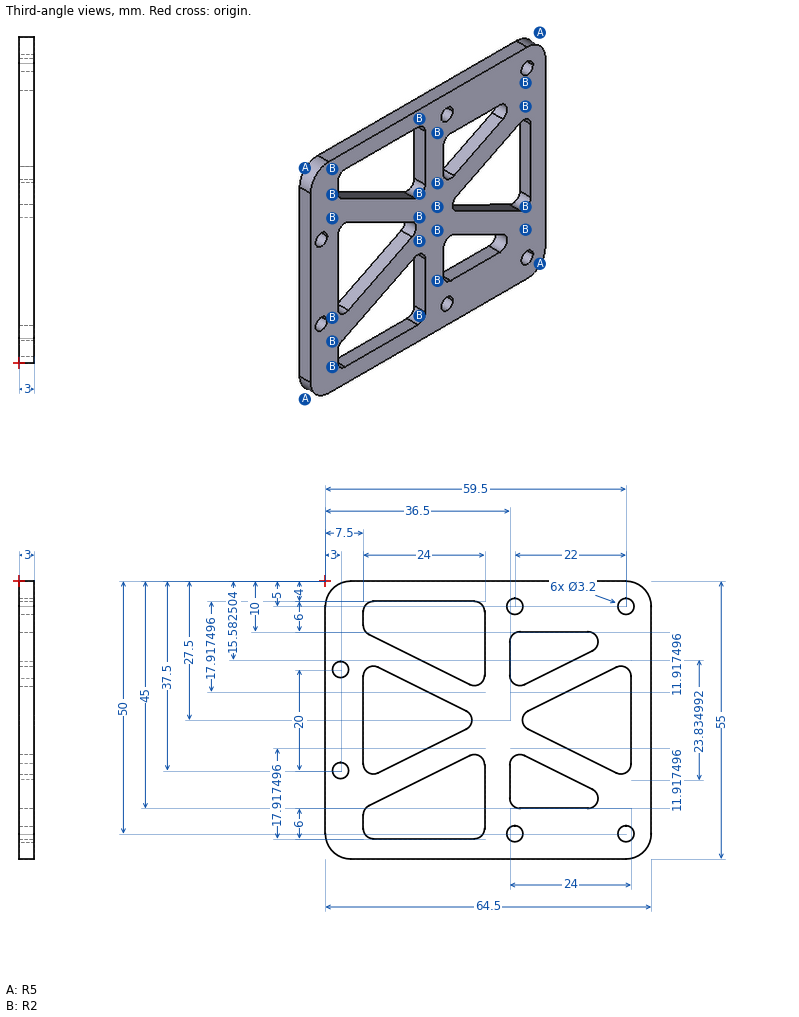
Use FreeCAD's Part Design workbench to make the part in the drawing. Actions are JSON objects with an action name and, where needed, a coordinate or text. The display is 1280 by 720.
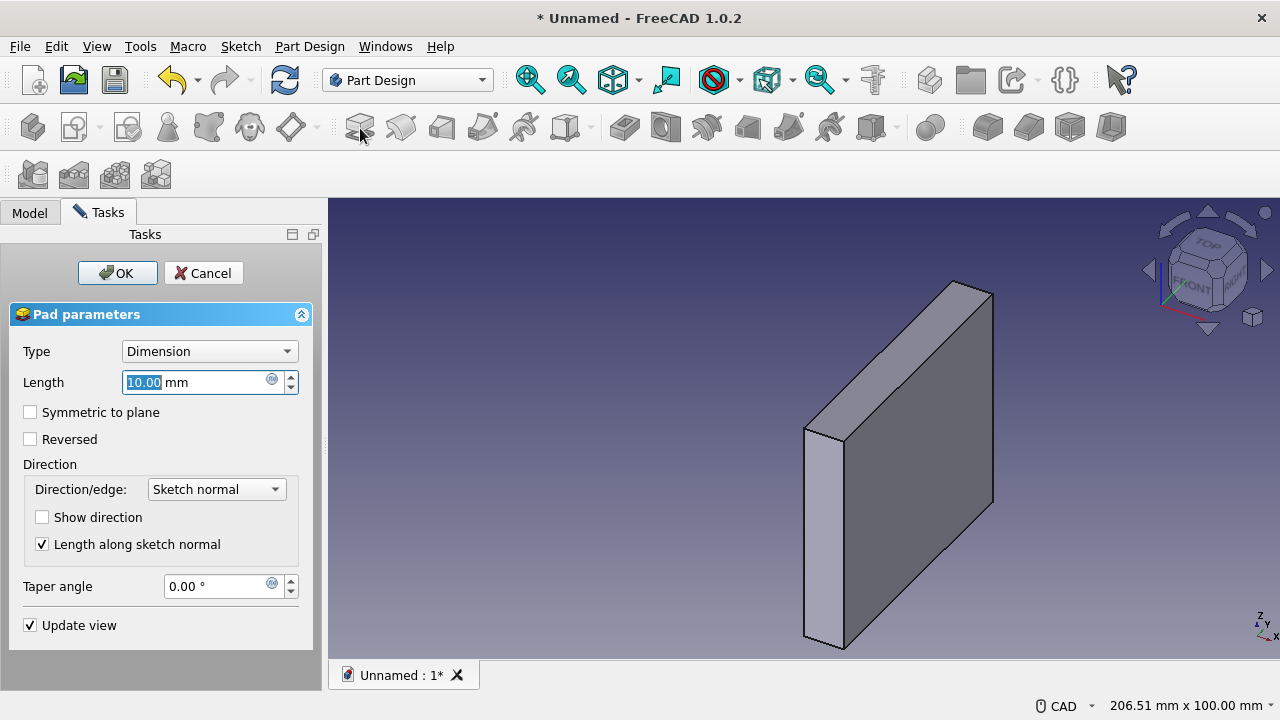
{"action": "type", "text": "3"}
{"action": "key", "text": "Tab"}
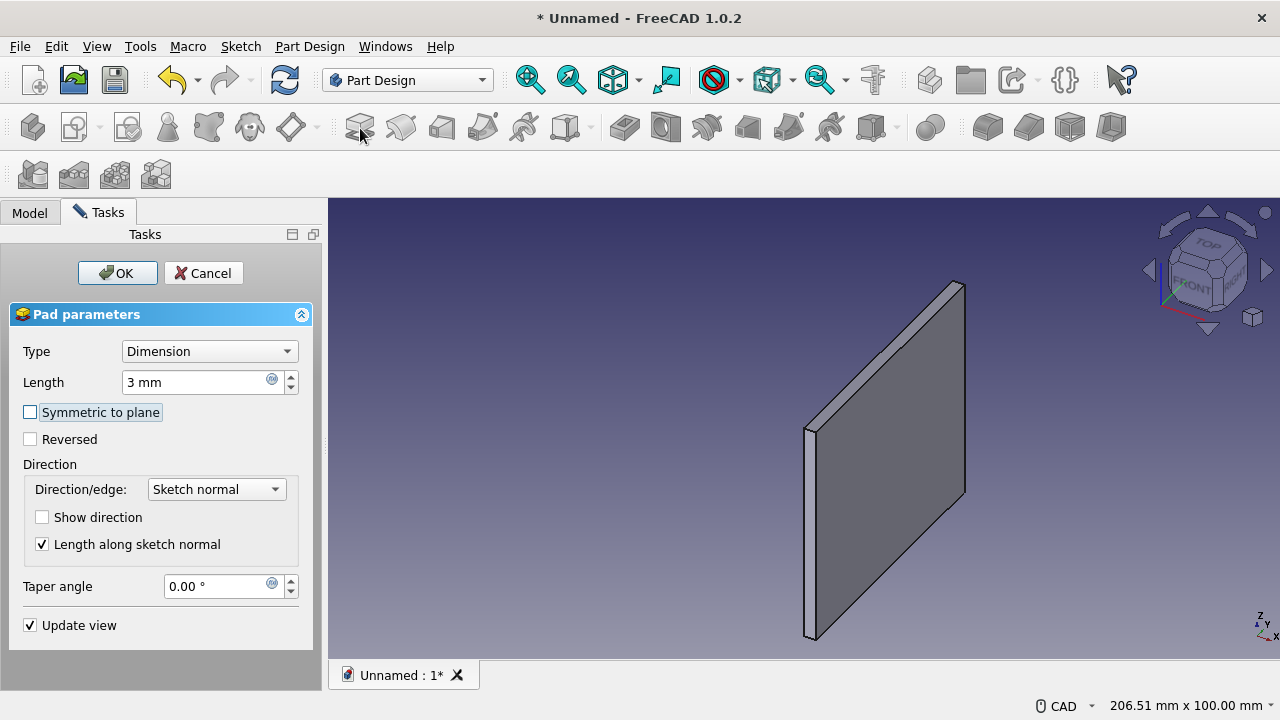
{"action": "left_click", "coordinate": [118, 273]}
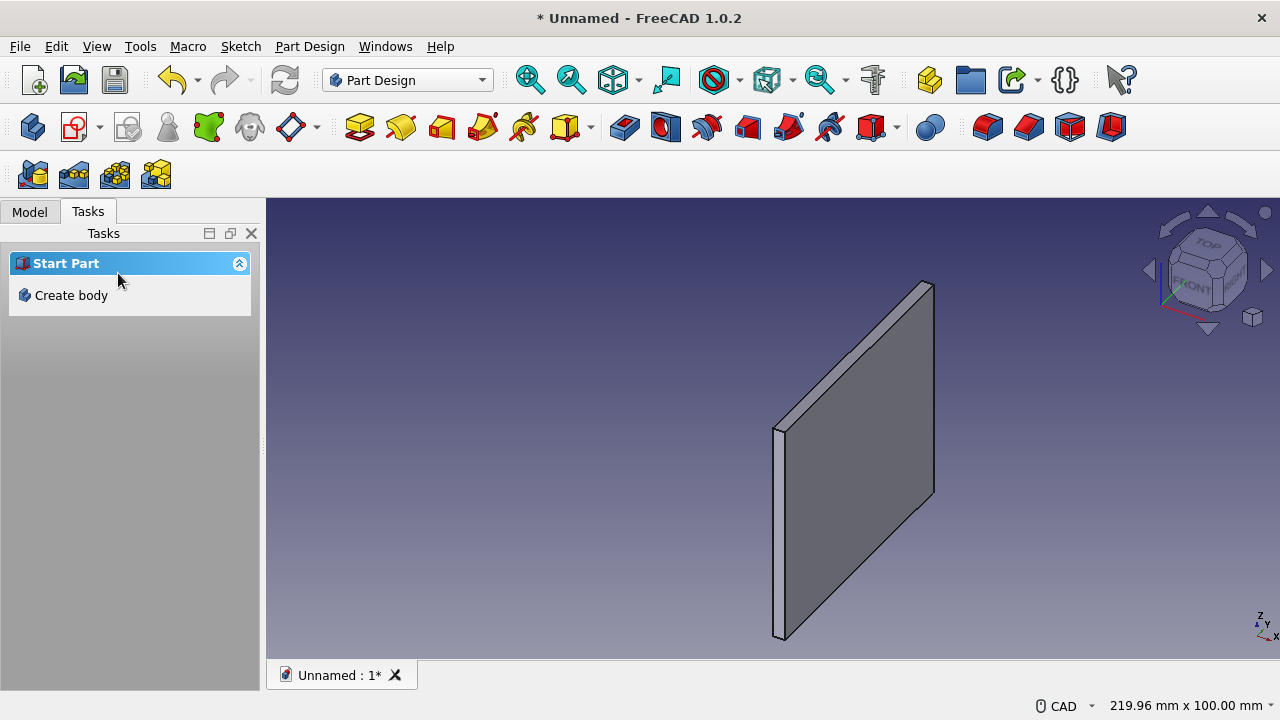
{"action": "left_click", "coordinate": [74, 128]}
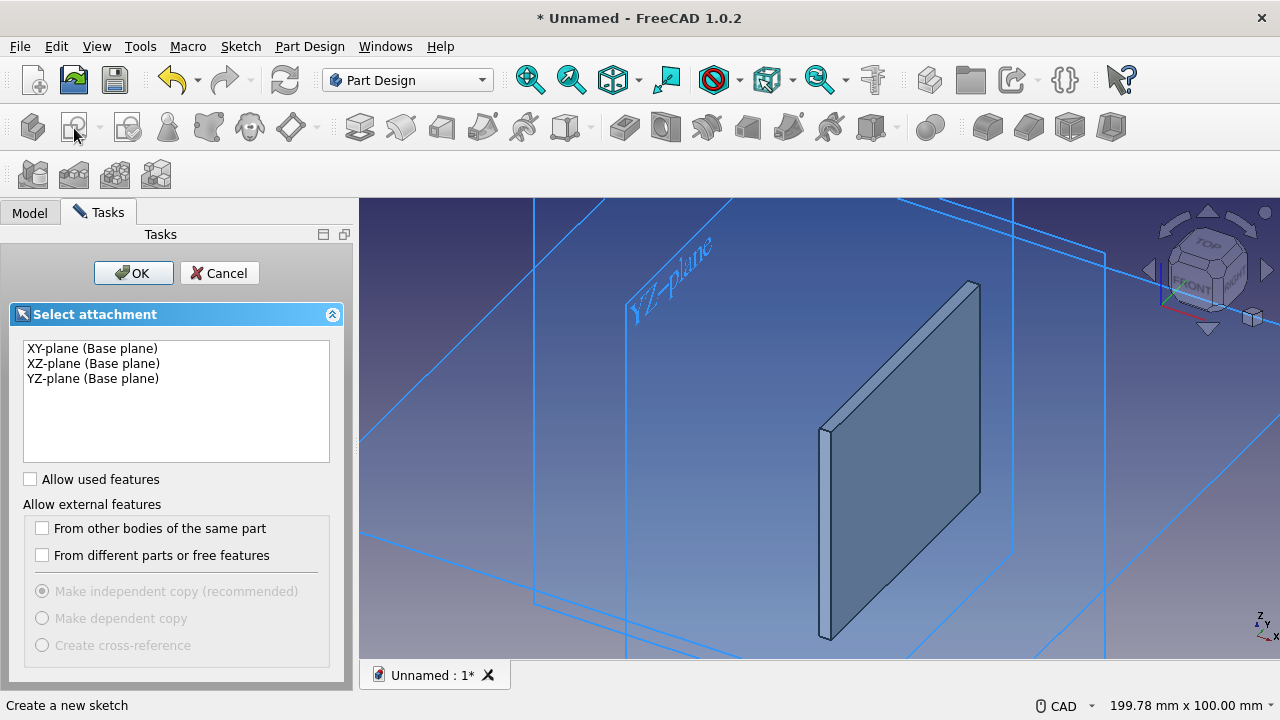
{"action": "left_click", "coordinate": [84, 378]}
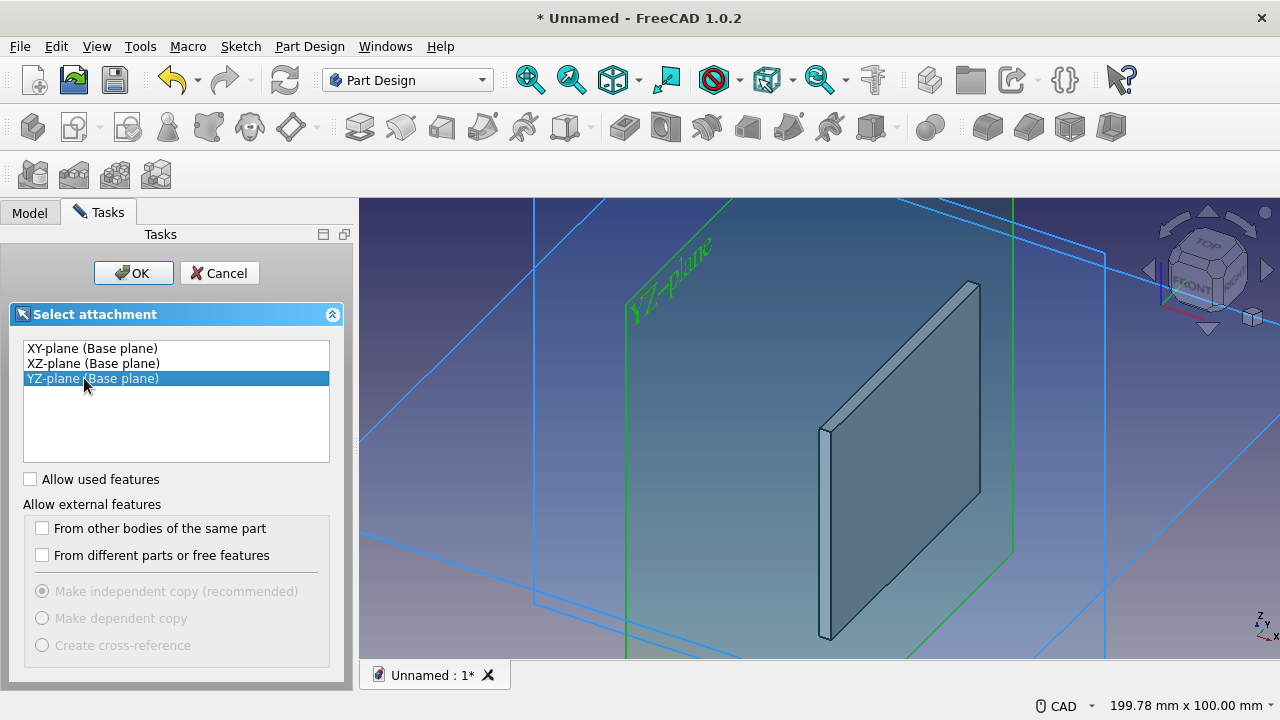
{"action": "left_click", "coordinate": [134, 273]}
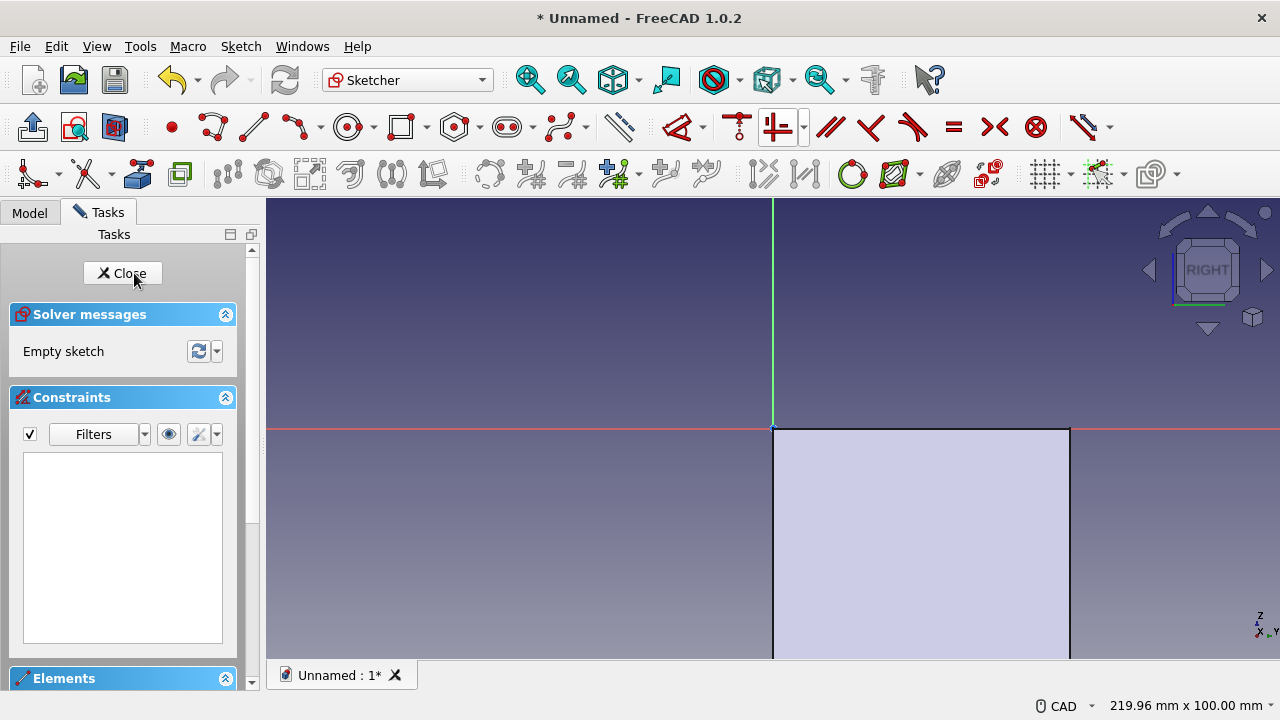
{"action": "left_click", "coordinate": [115, 128]}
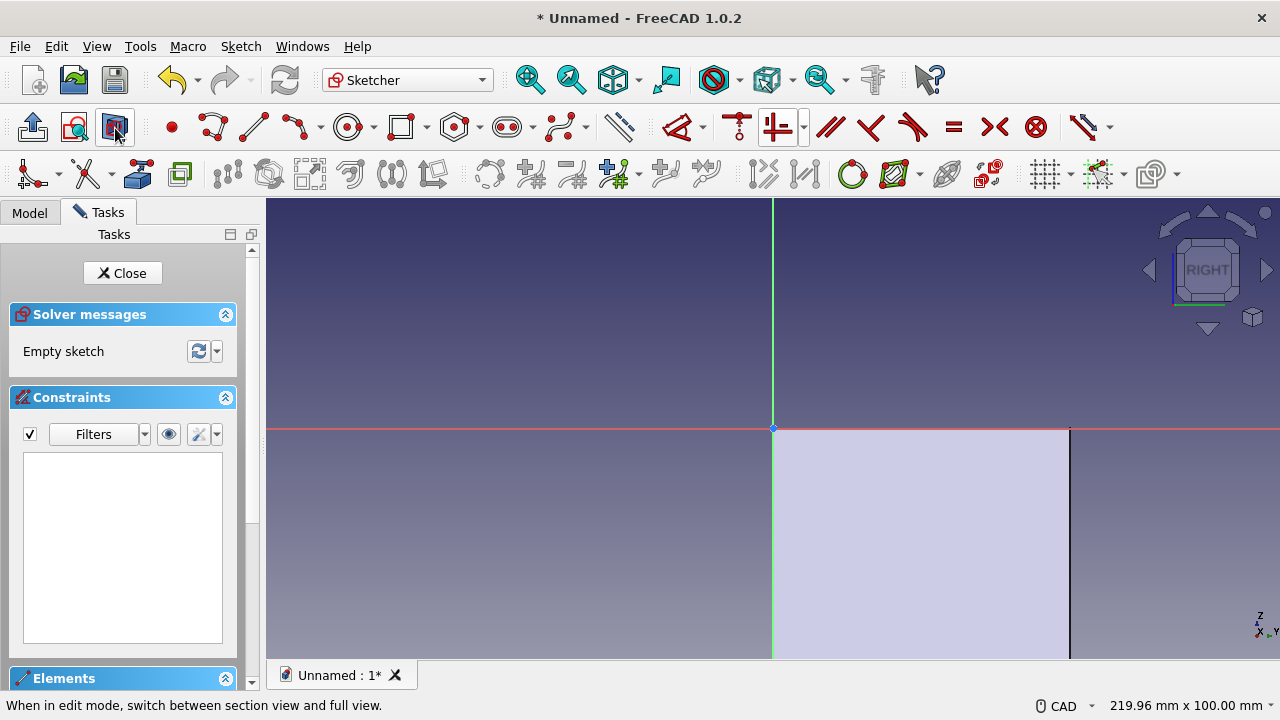
{"action": "scroll", "coordinate": [294, 226], "scroll_direction": "down", "scroll_amount": 1}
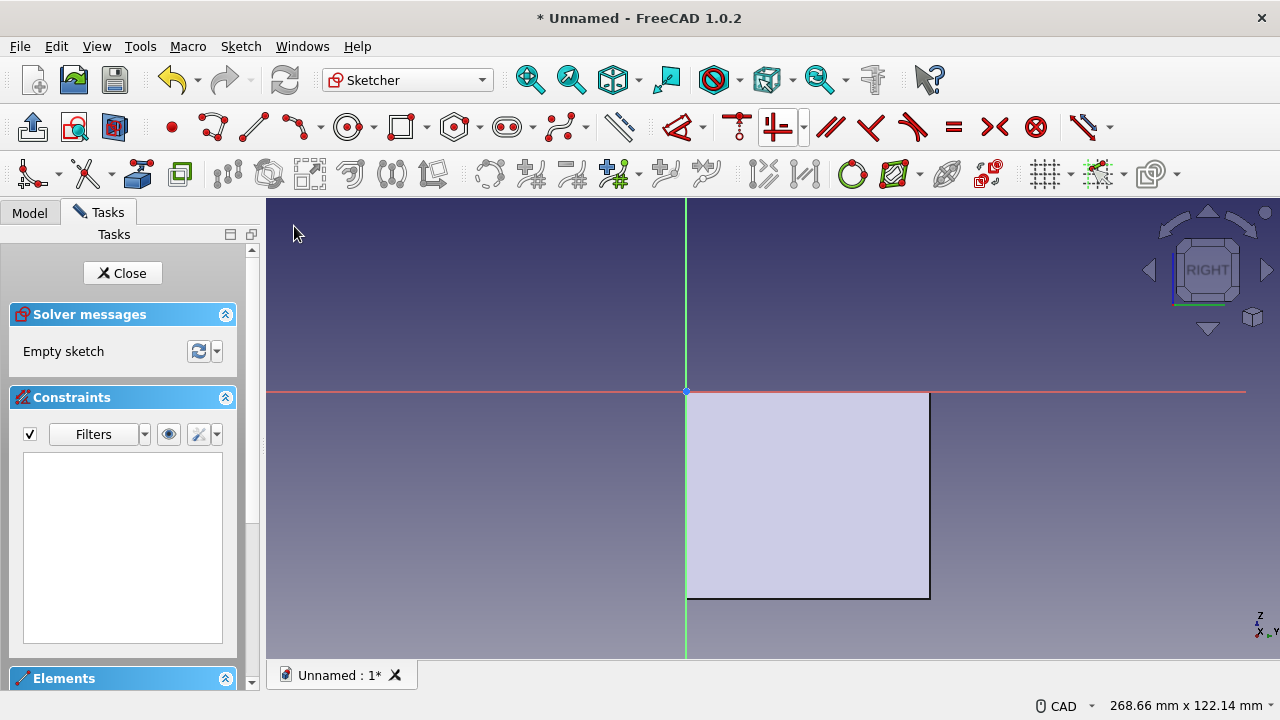
{"action": "scroll", "coordinate": [999, 613], "scroll_direction": "up", "scroll_amount": 2}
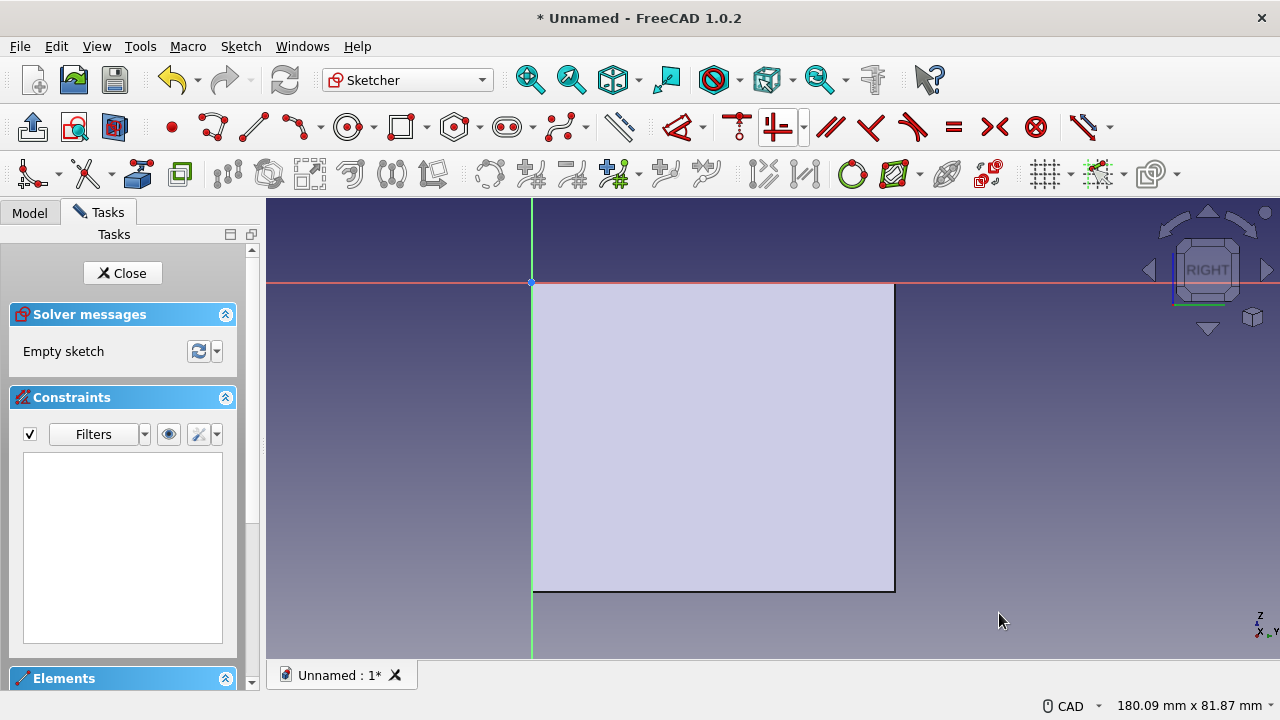
{"action": "left_click", "coordinate": [348, 128]}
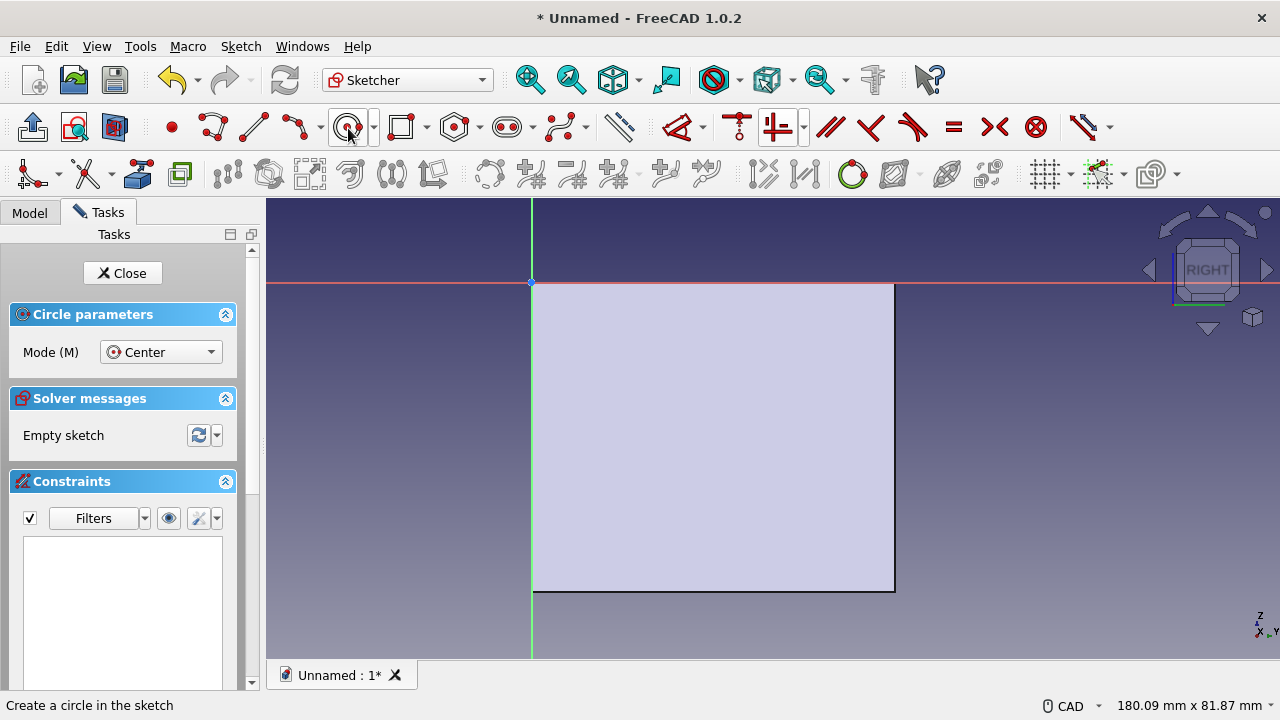
{"action": "scroll", "coordinate": [867, 311], "scroll_direction": "up", "scroll_amount": 5}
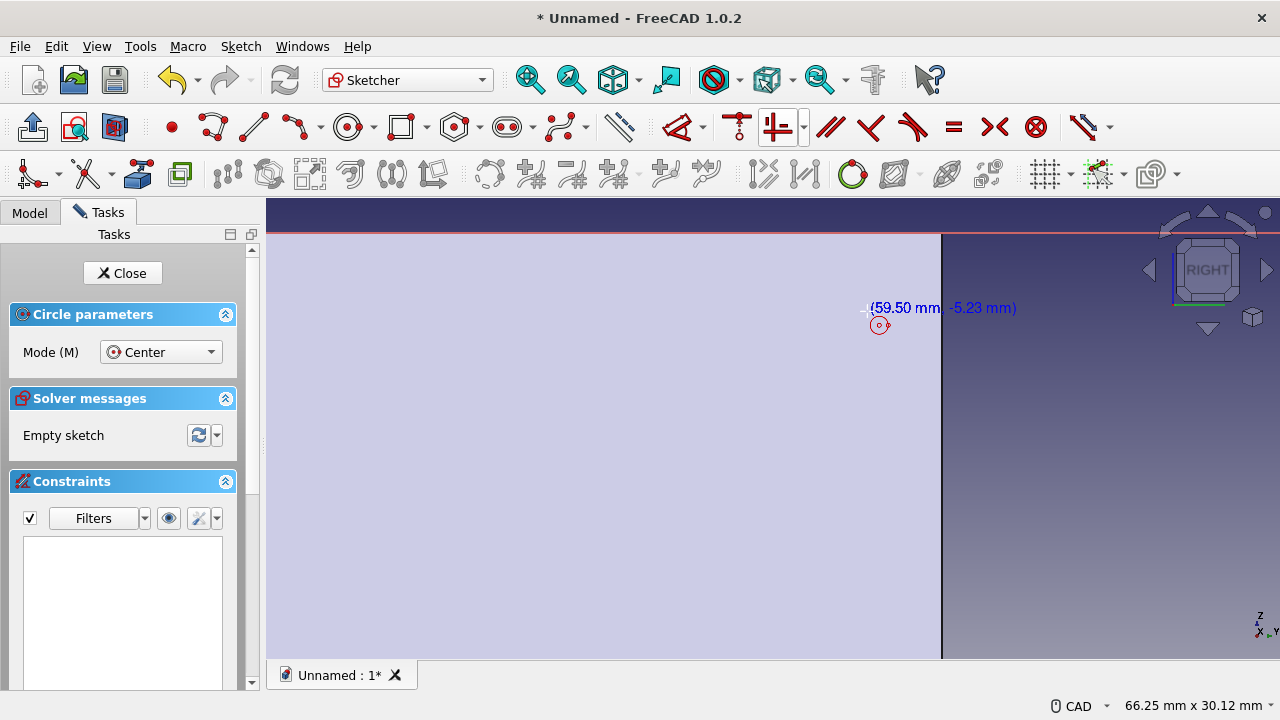
{"action": "left_click", "coordinate": [866, 310]}
{"action": "mouse_move", "coordinate": [883, 293]}